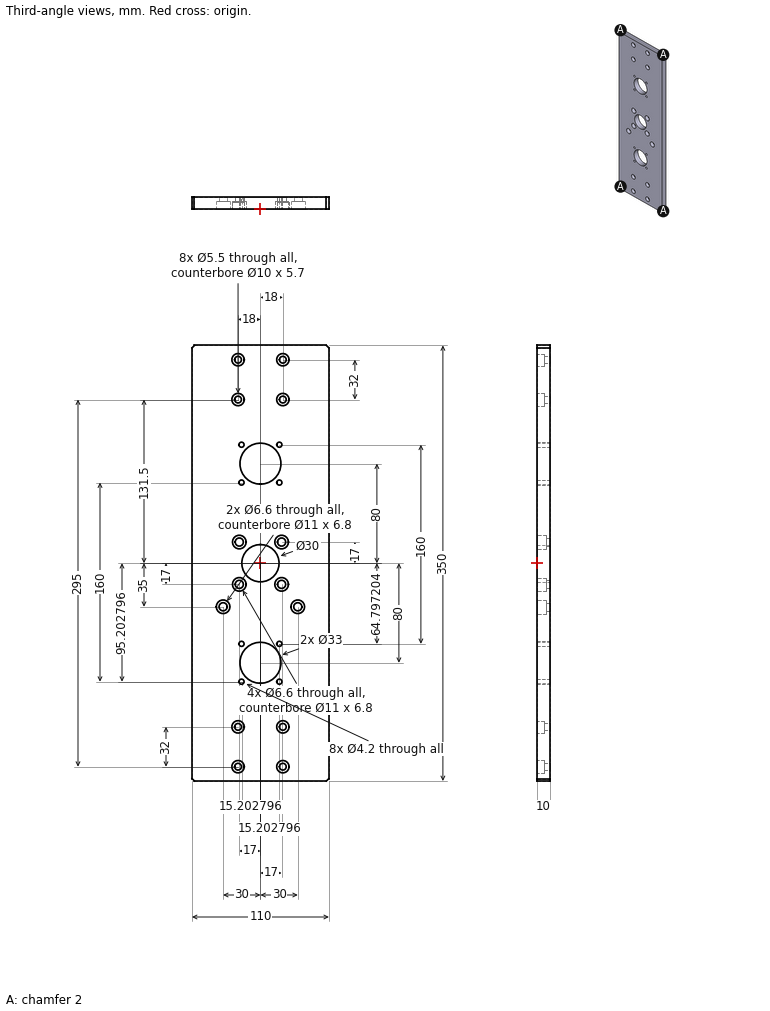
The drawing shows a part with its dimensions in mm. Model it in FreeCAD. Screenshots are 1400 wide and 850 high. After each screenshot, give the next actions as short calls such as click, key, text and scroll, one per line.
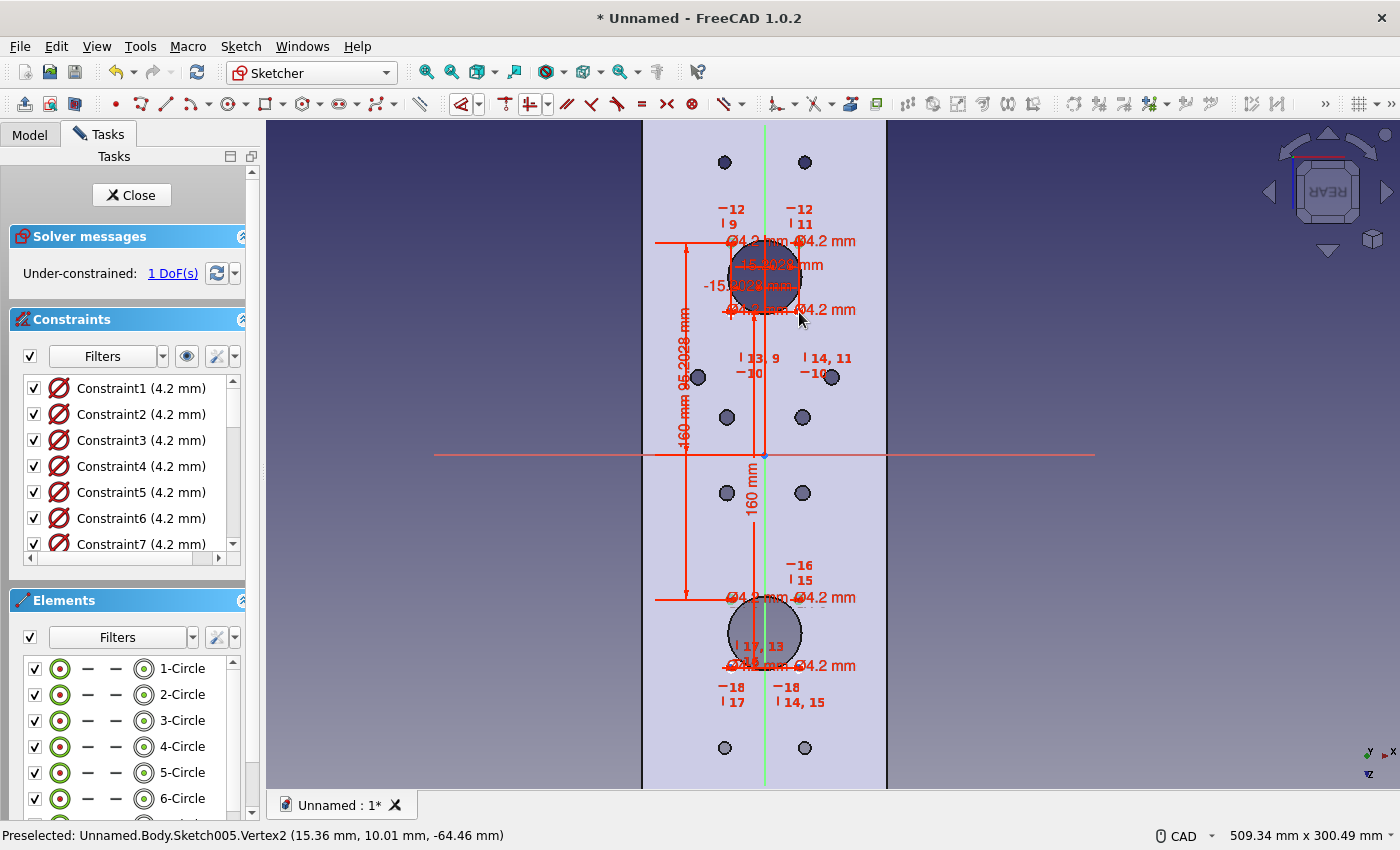
click(799, 312)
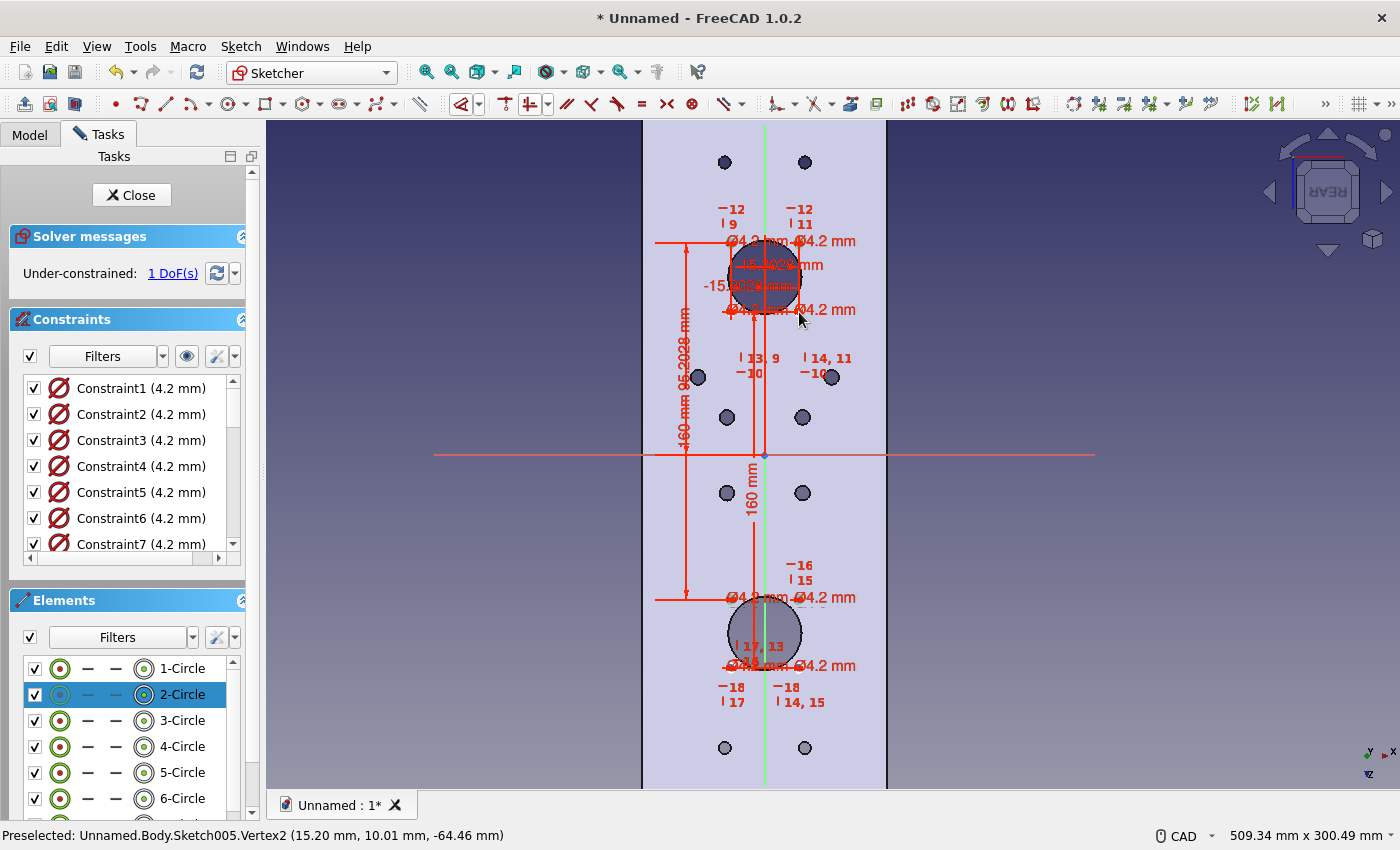
key(i)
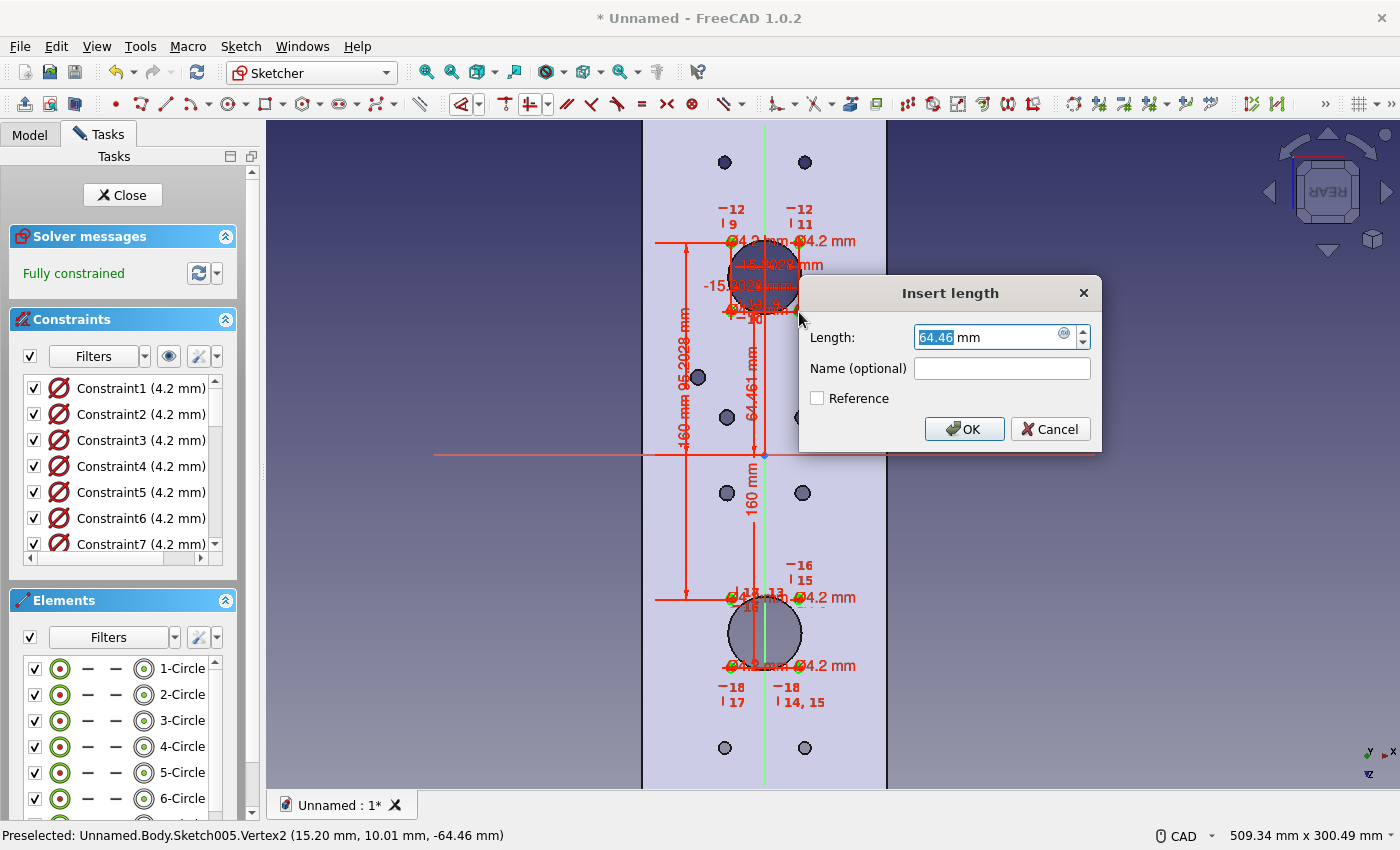
text(64.797204)
key(Return)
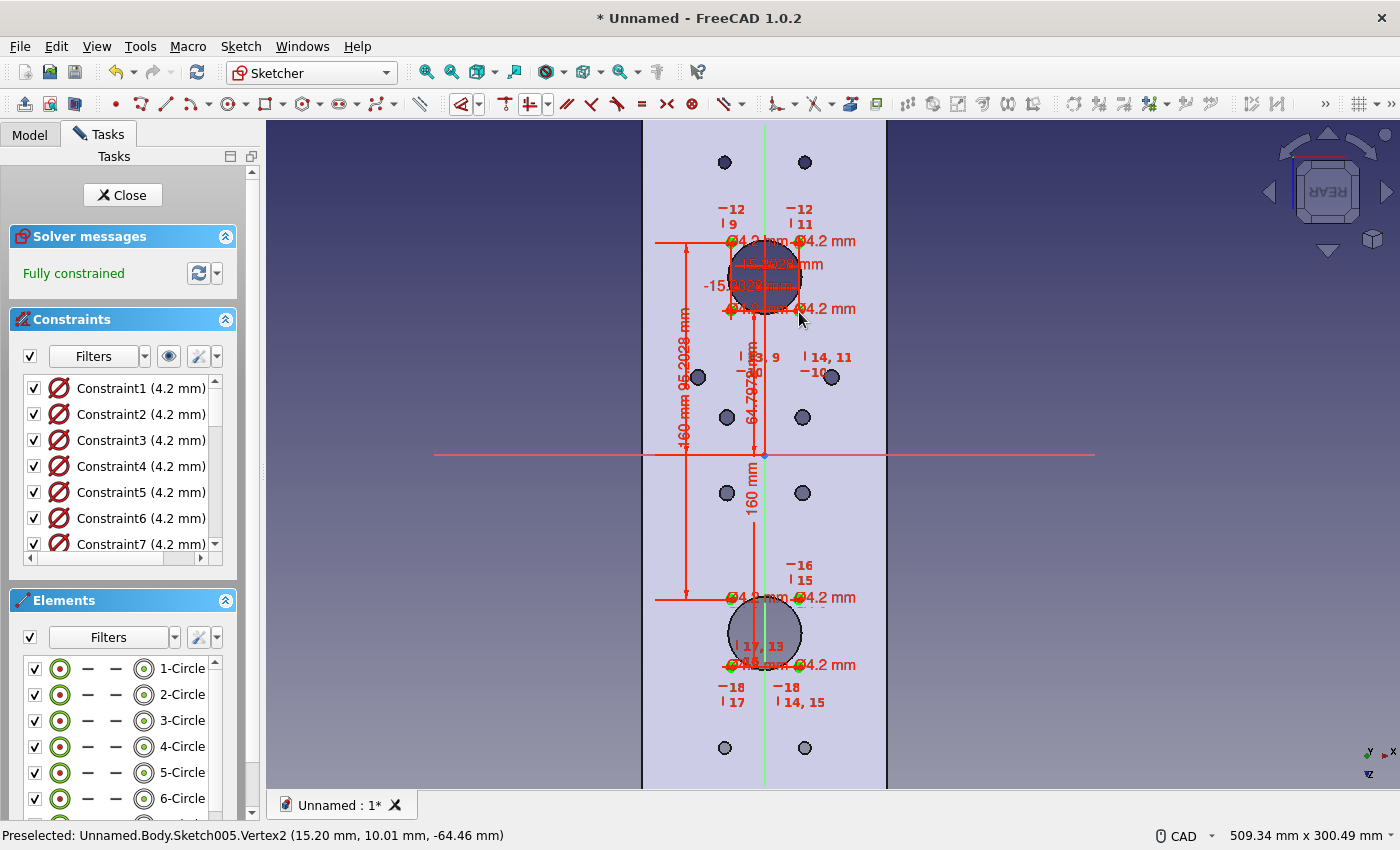
click(123, 195)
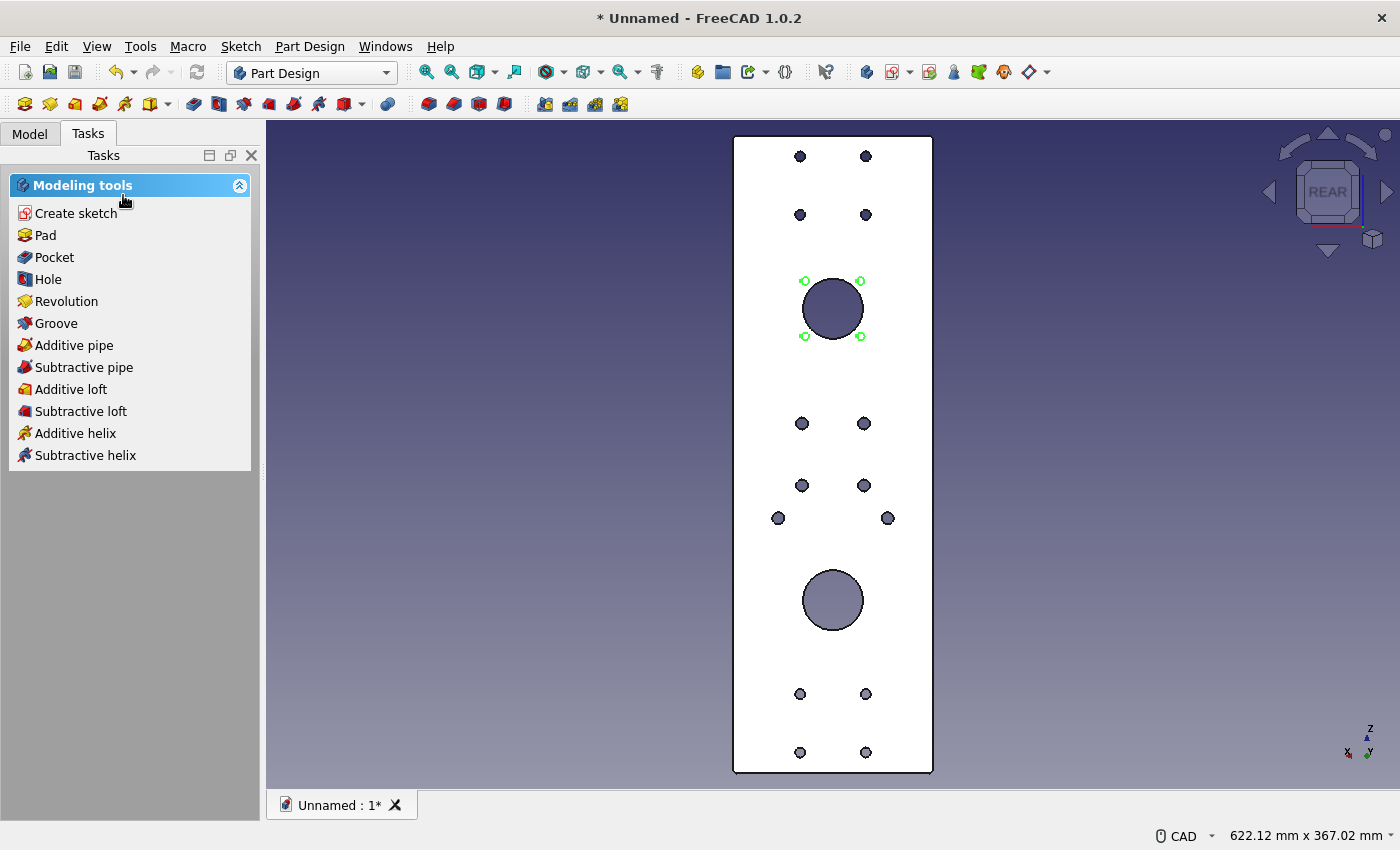
click(219, 104)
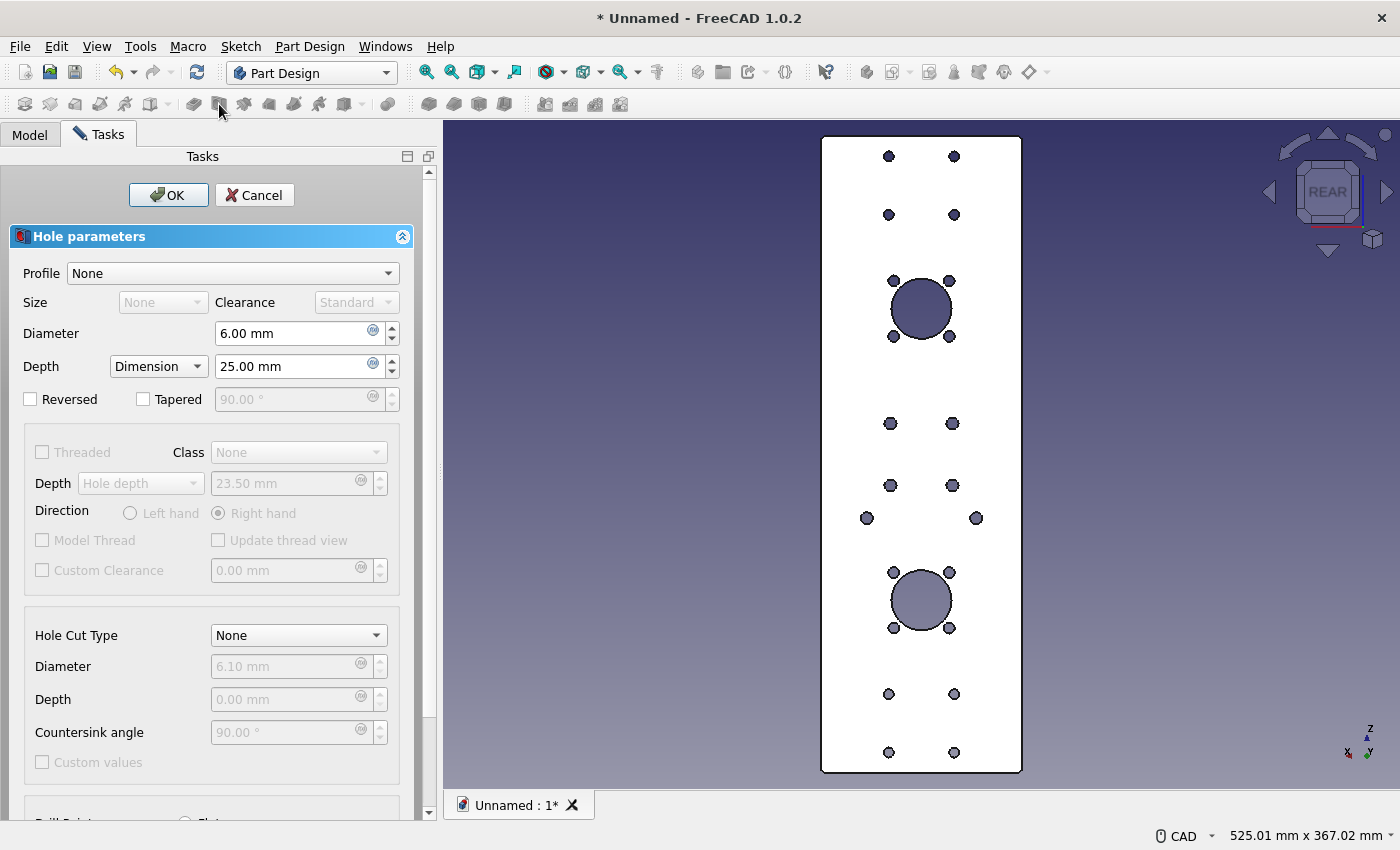
triple_click(300, 334)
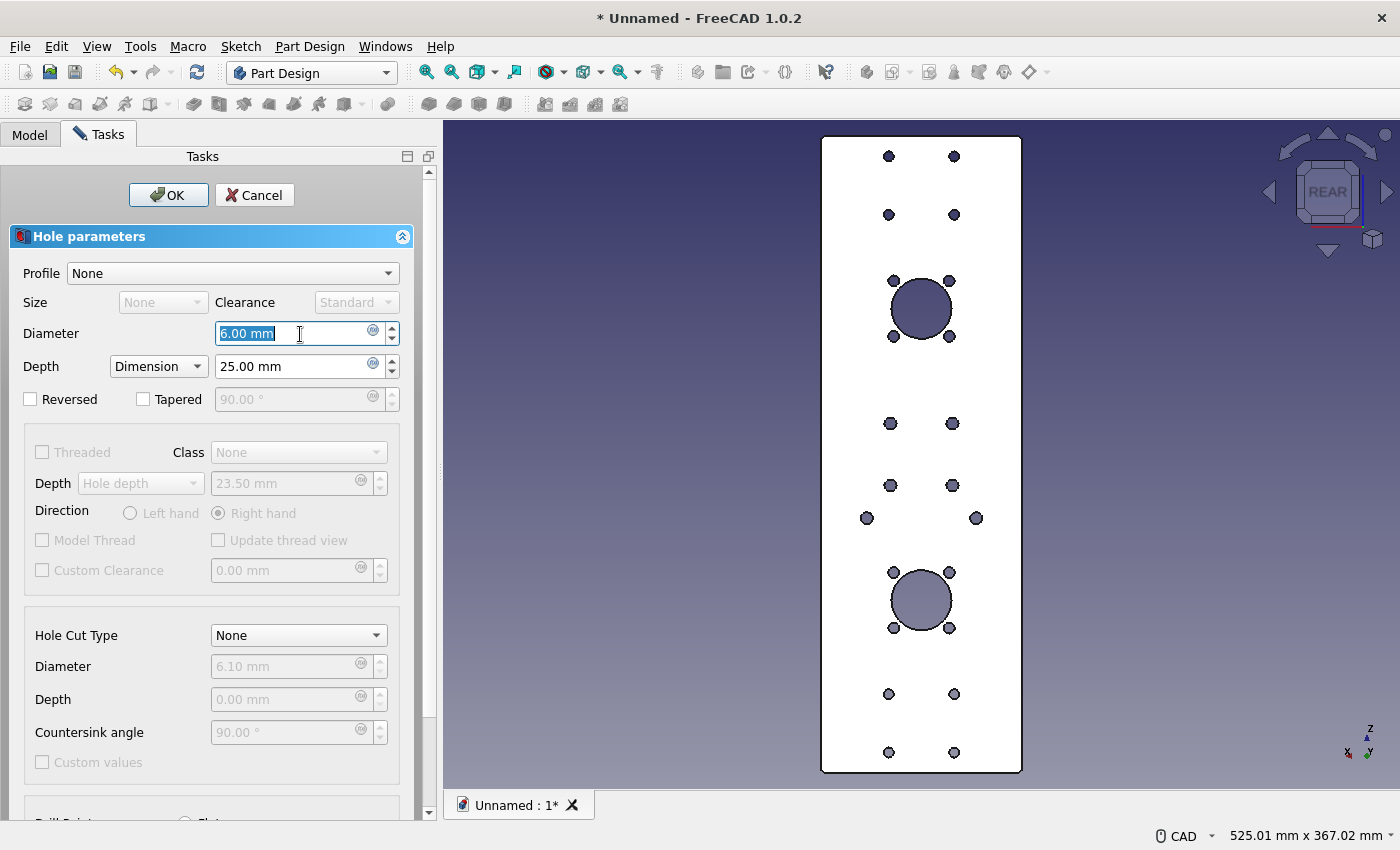
text(4.2)
key(Tab)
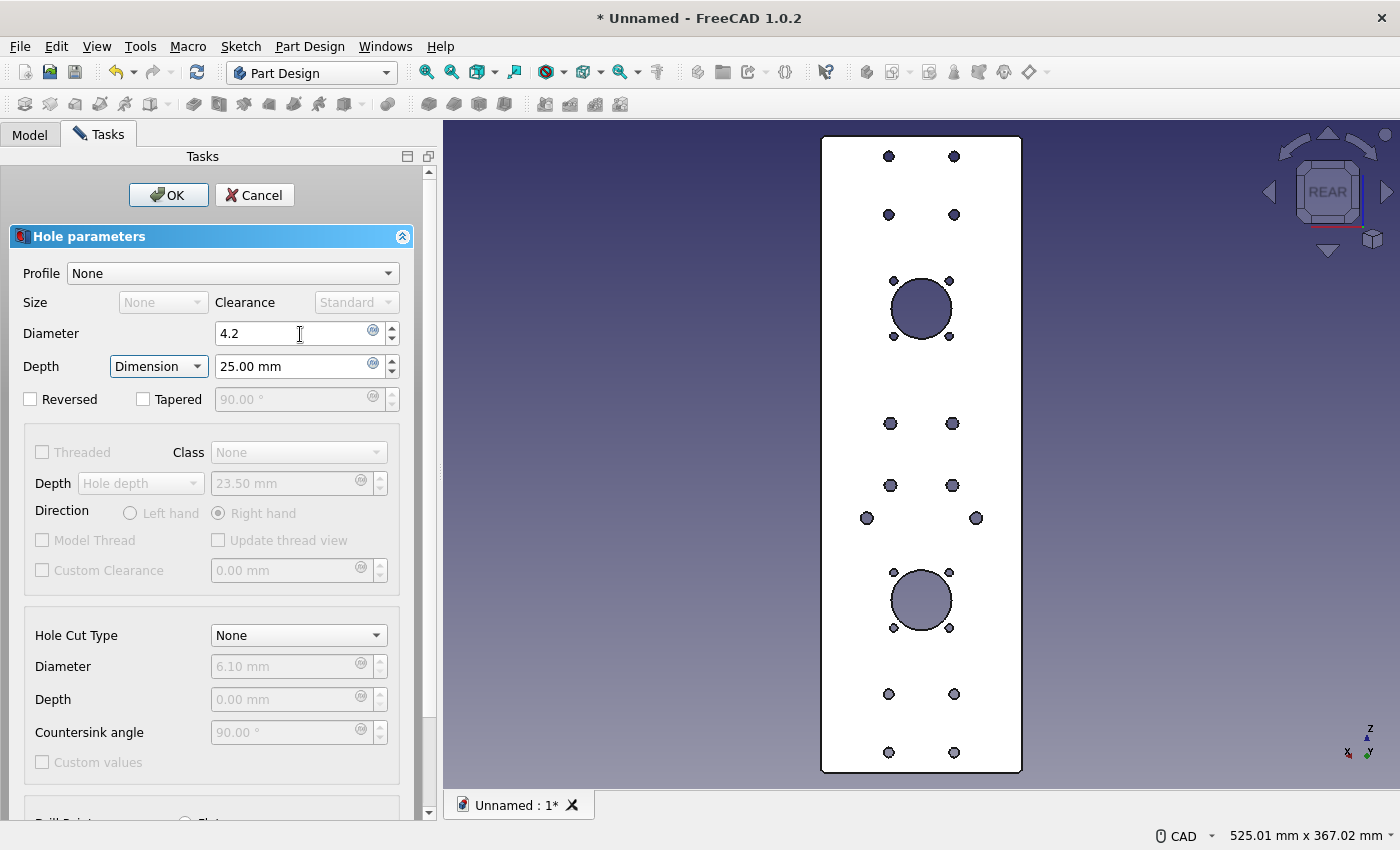
click(160, 366)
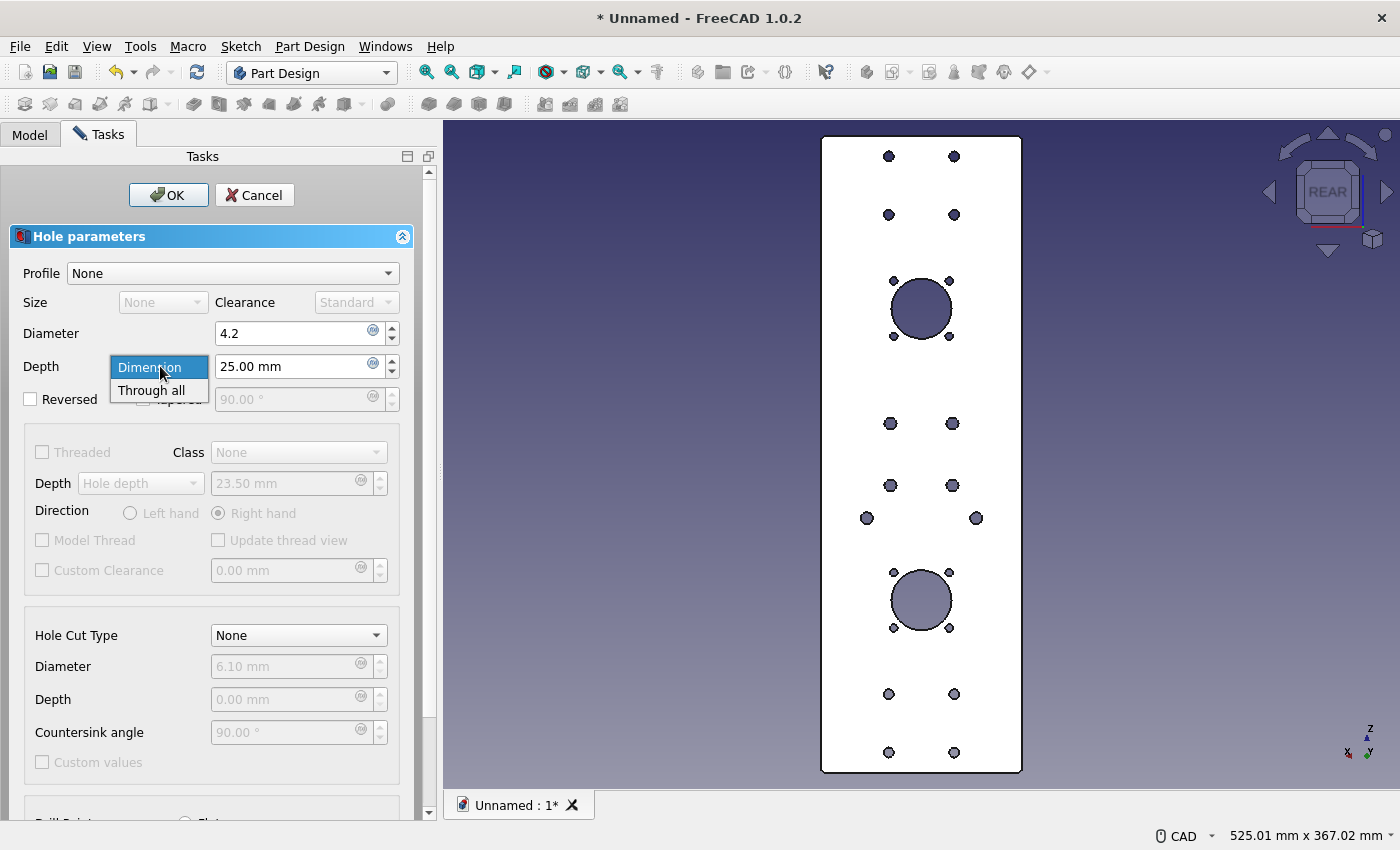
click(158, 390)